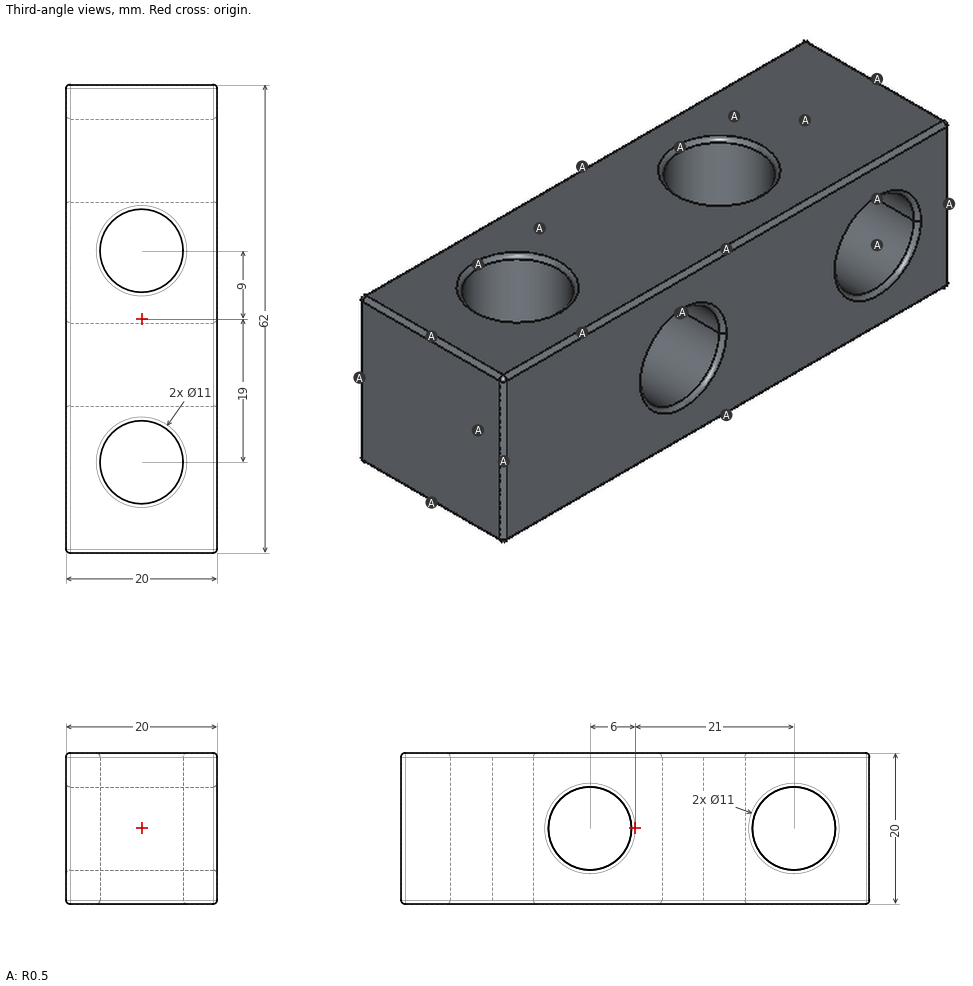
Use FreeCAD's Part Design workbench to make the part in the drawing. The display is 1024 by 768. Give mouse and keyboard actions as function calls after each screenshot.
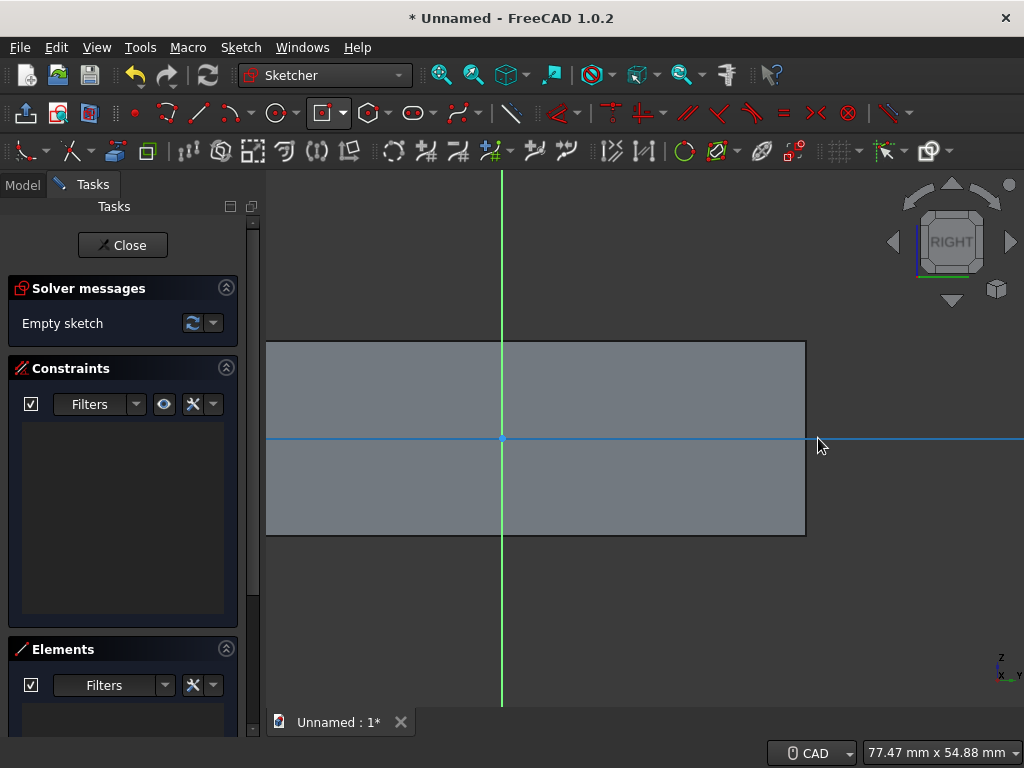
click(276, 114)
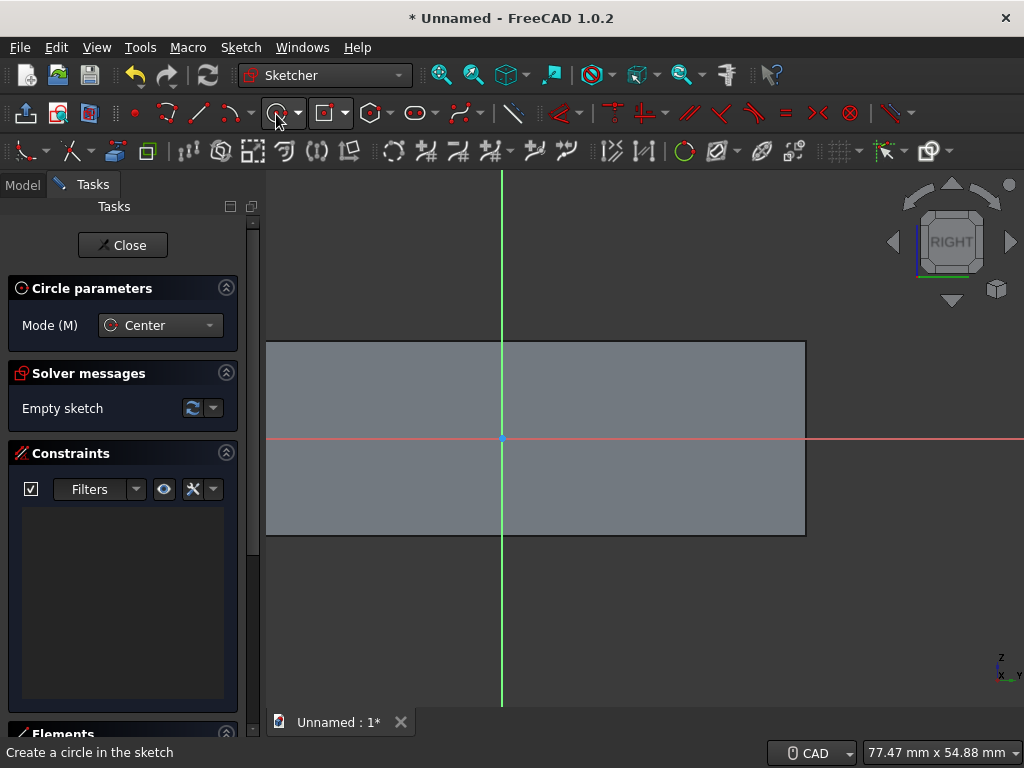
click(708, 438)
move(746, 400)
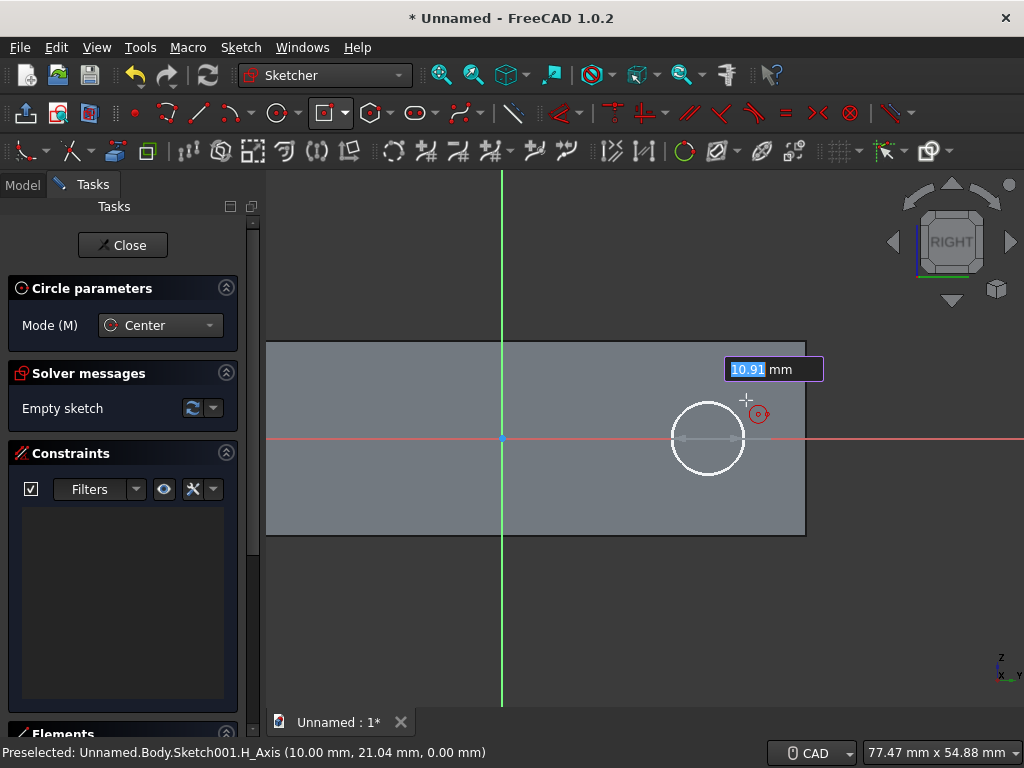
text(11)
key(Return)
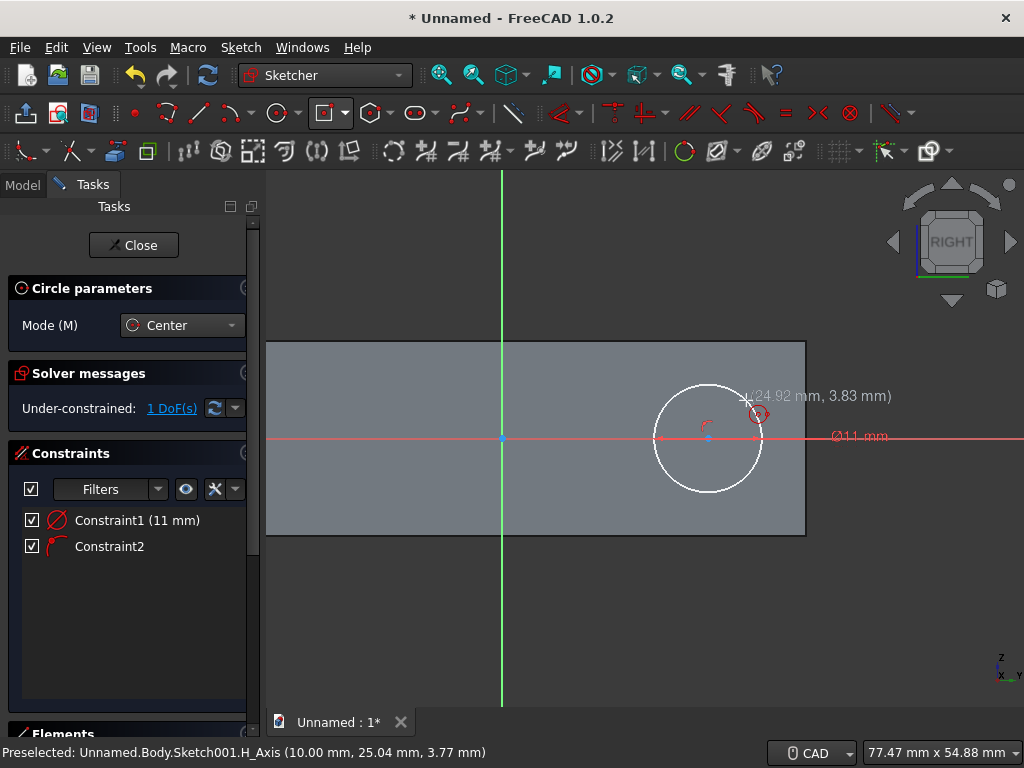
click(443, 438)
move(482, 400)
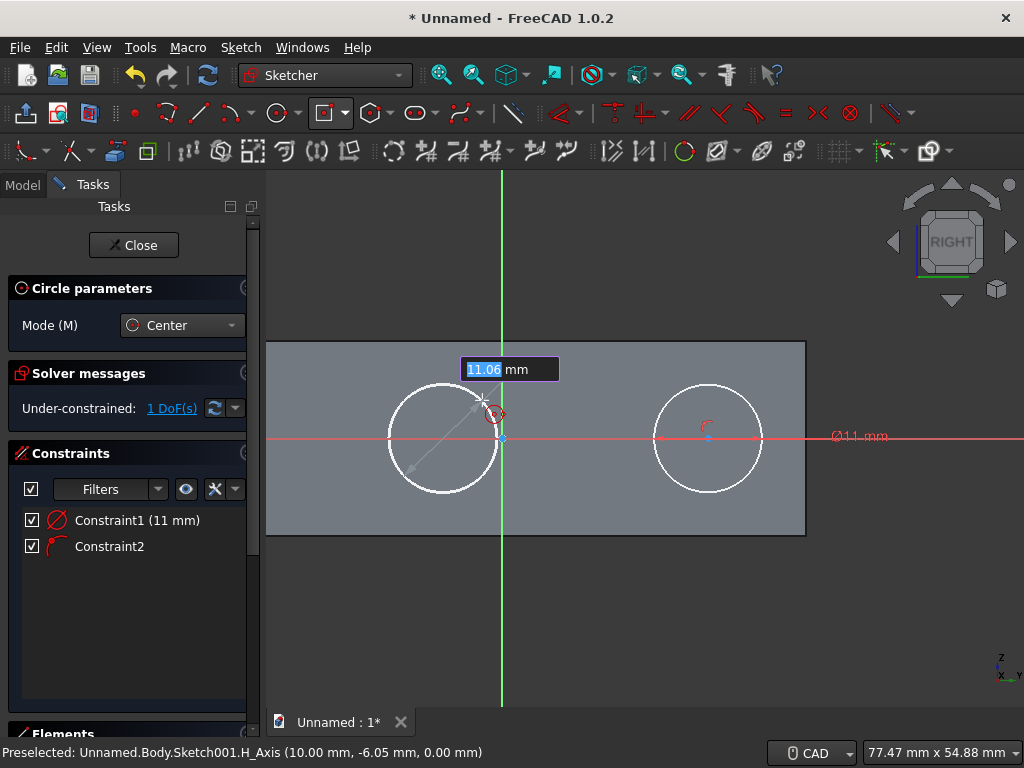
text(11)
key(Return)
key(Escape)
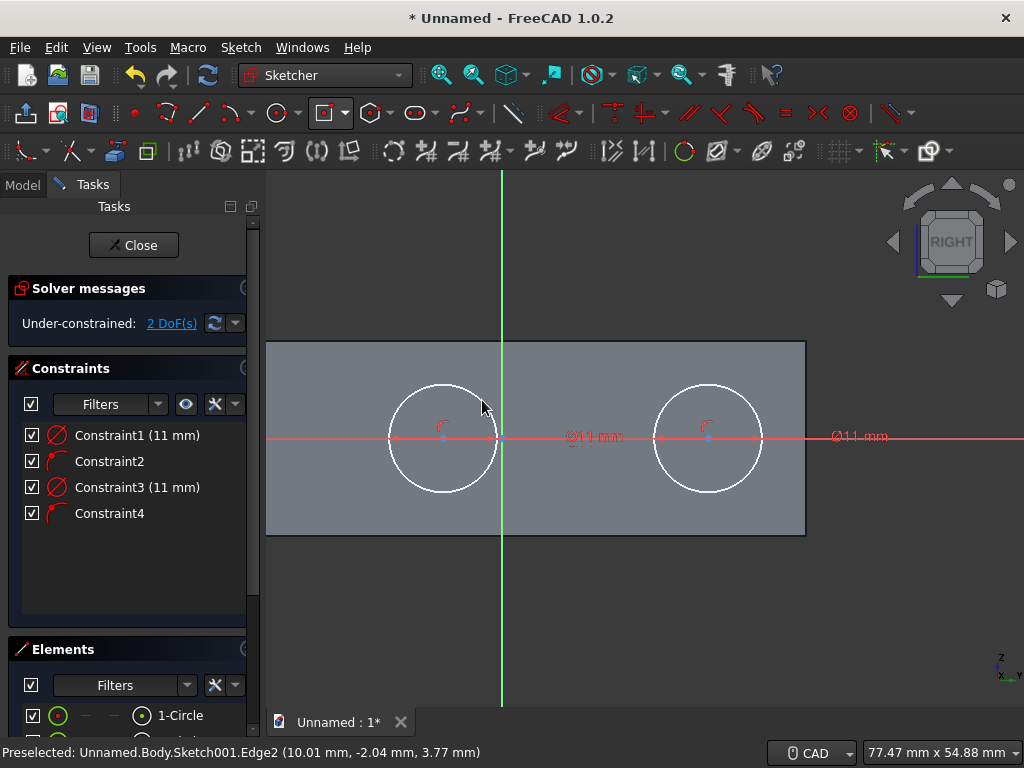
key(d)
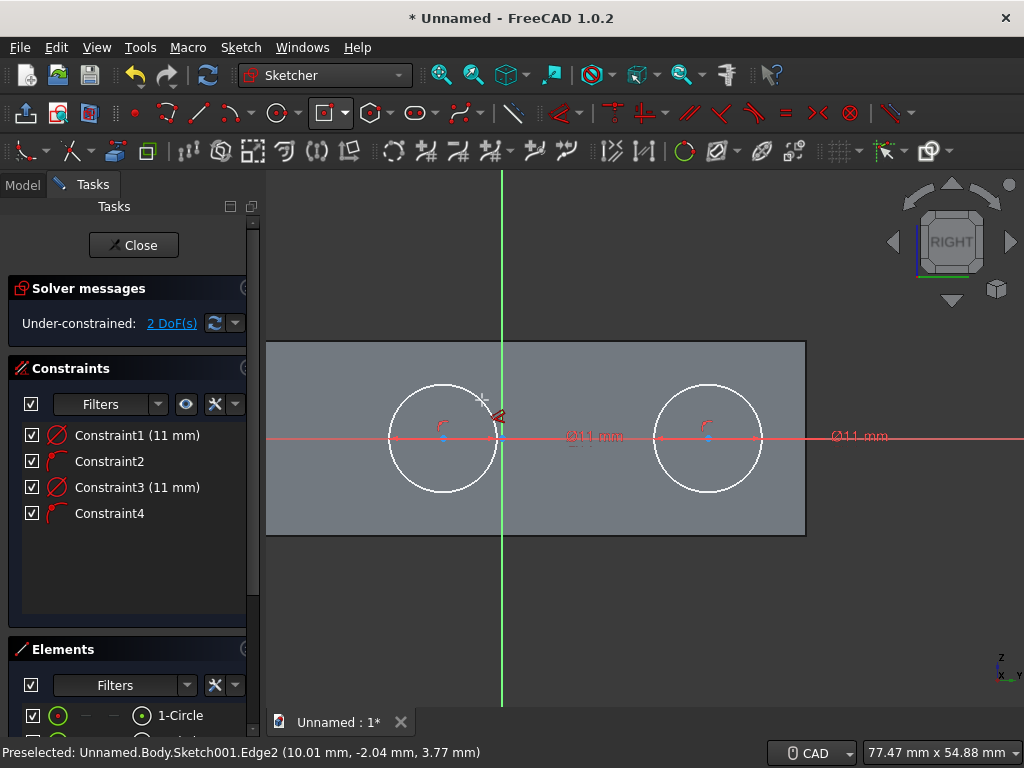
click(443, 438)
click(459, 472)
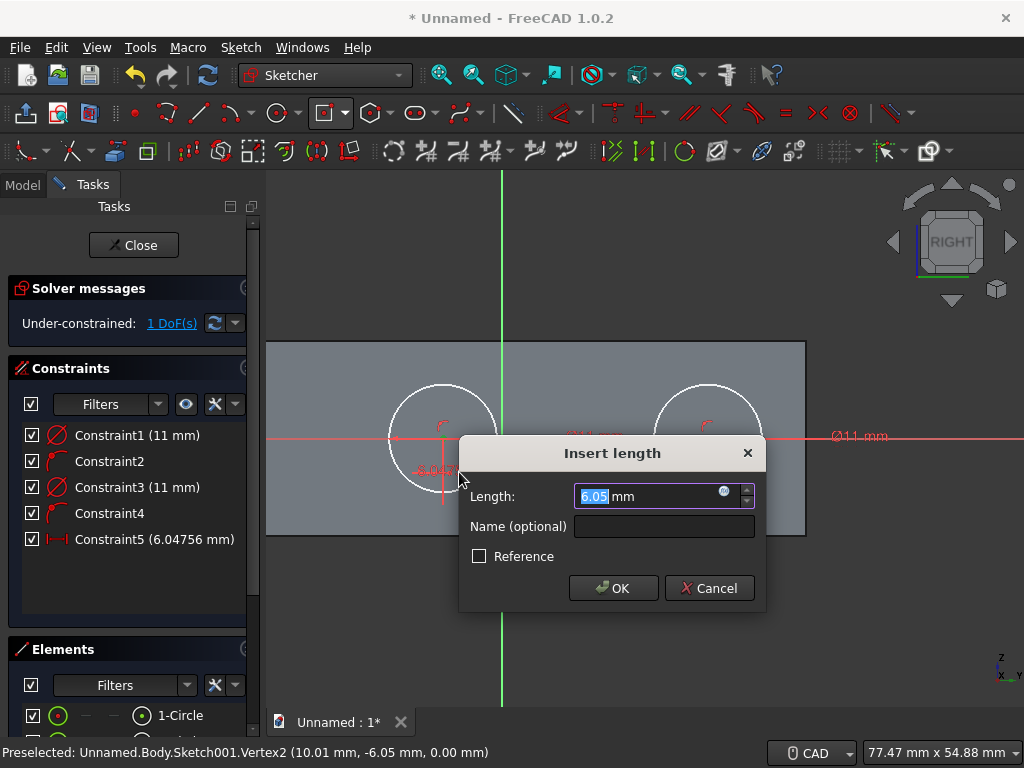
text(6)
key(Return)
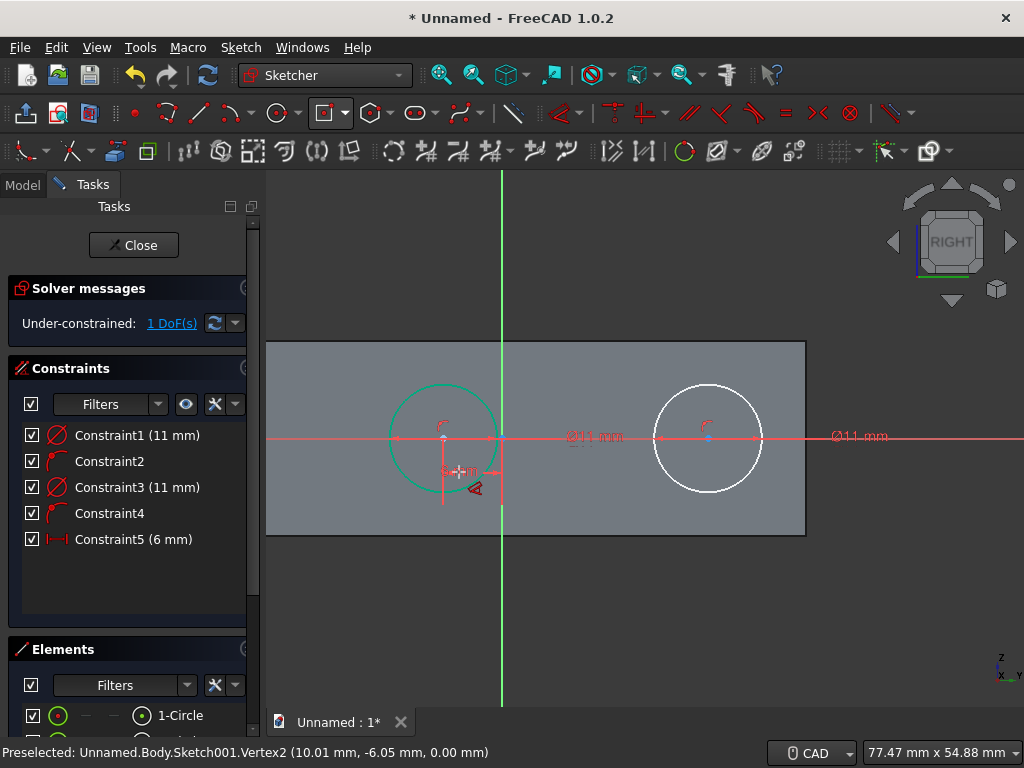
click(708, 438)
click(605, 472)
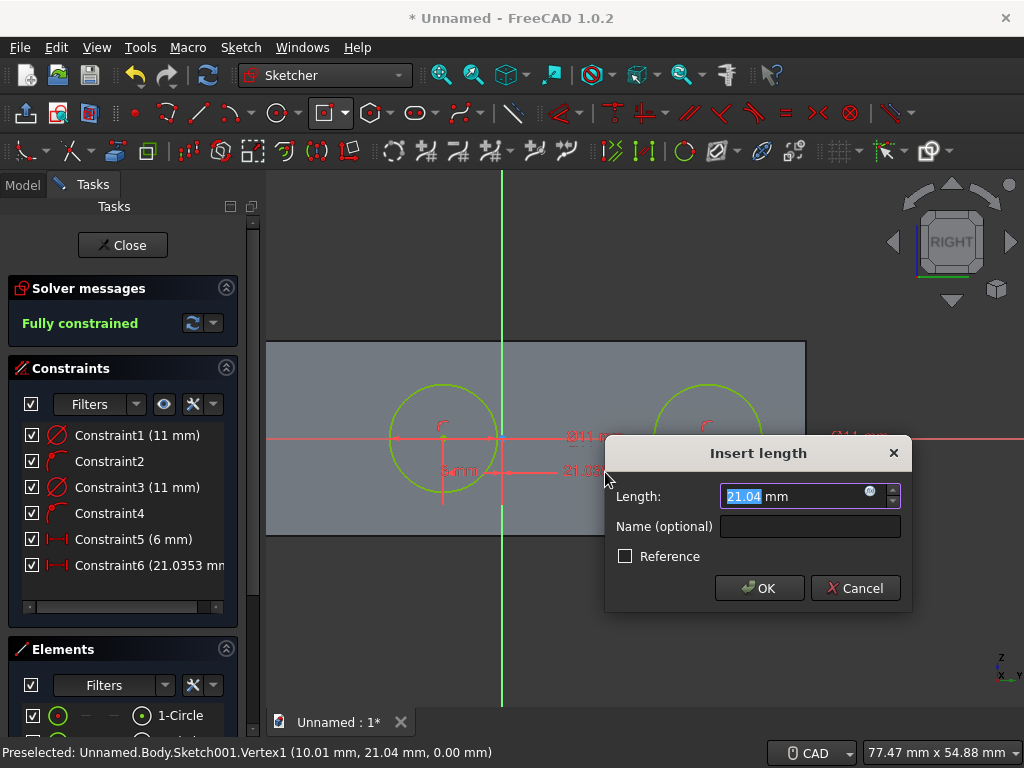
text(21)
key(Return)
key(Escape)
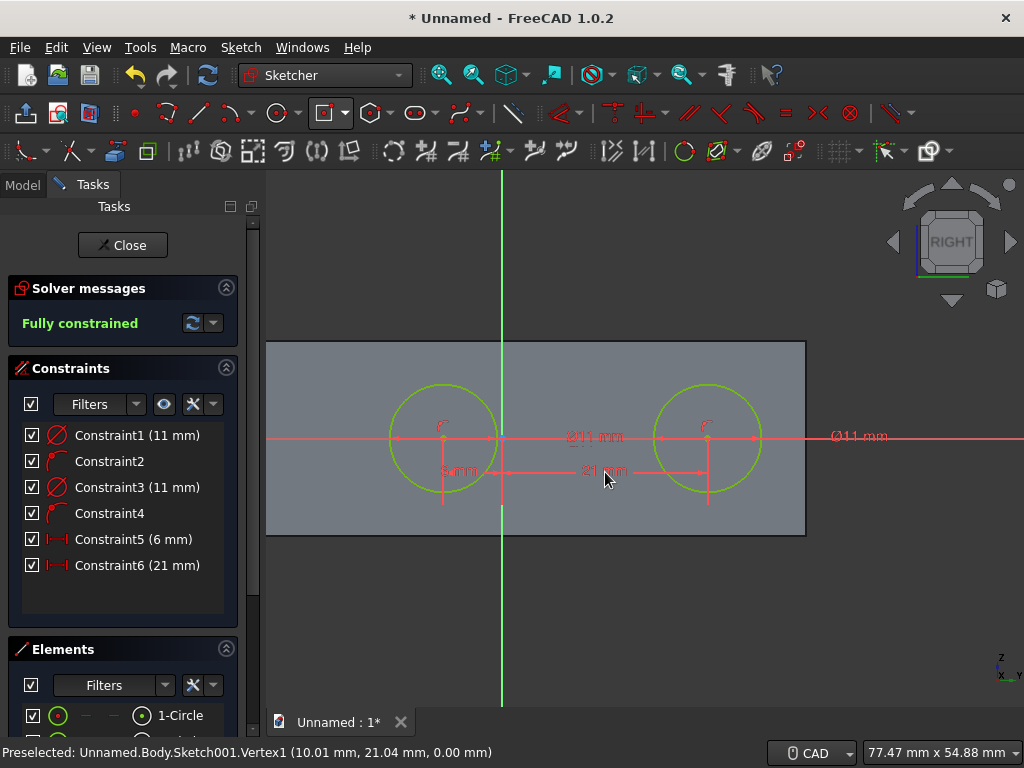
click(123, 245)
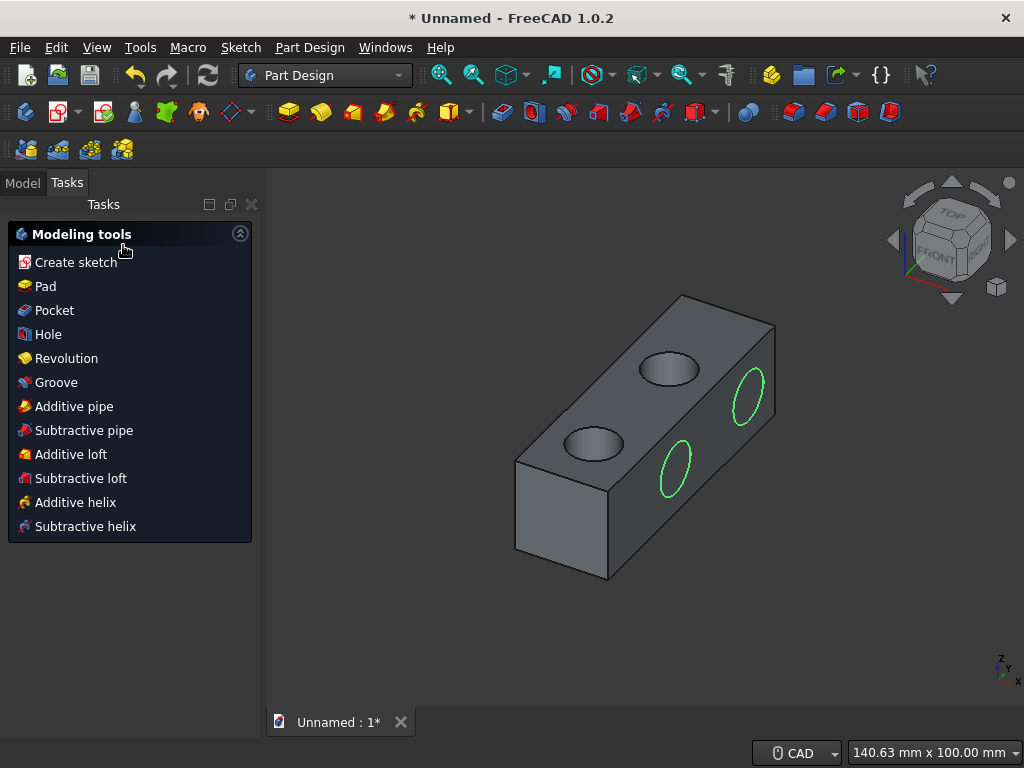
click(504, 112)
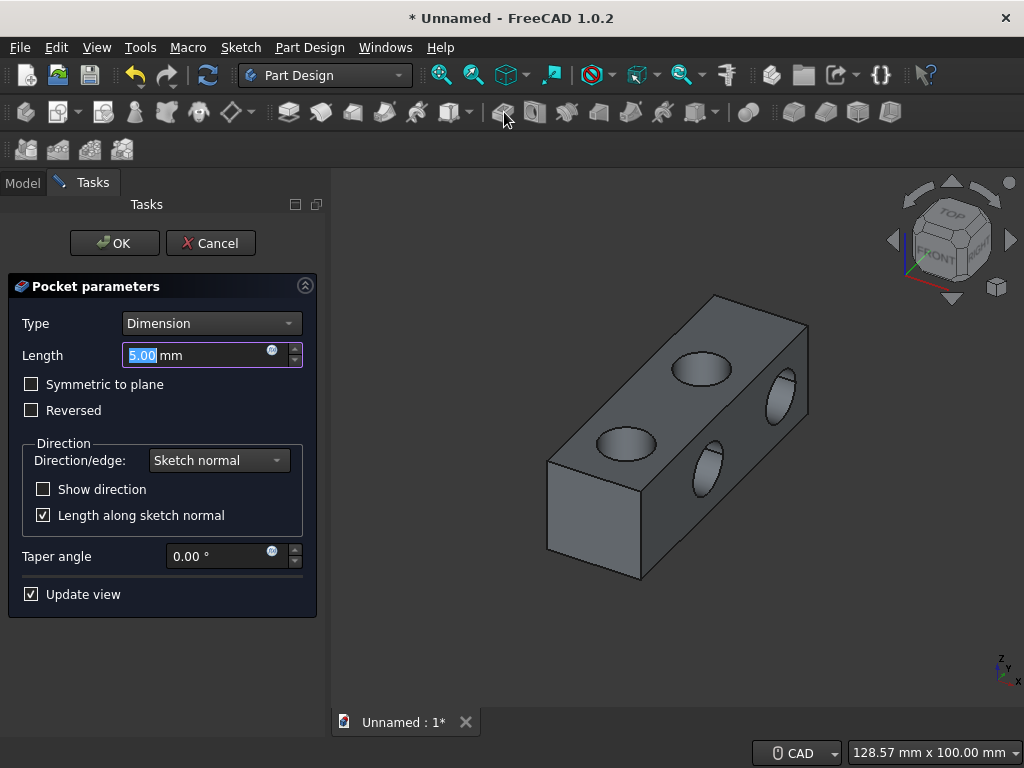
text(20)
key(Tab)